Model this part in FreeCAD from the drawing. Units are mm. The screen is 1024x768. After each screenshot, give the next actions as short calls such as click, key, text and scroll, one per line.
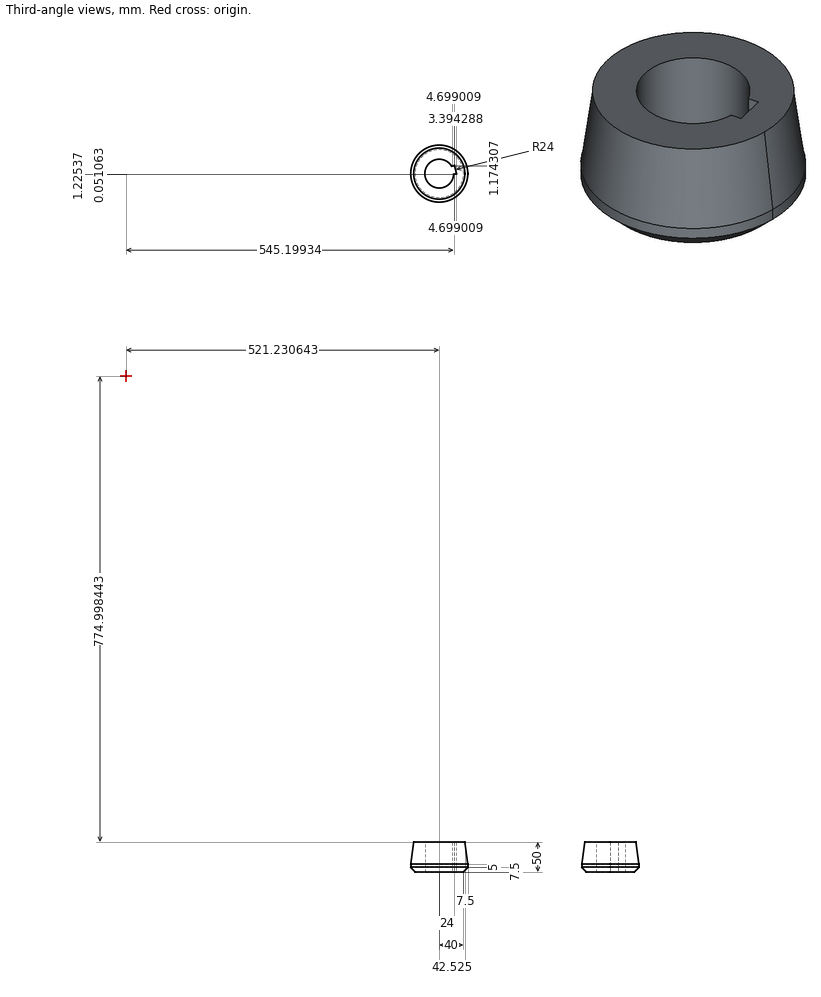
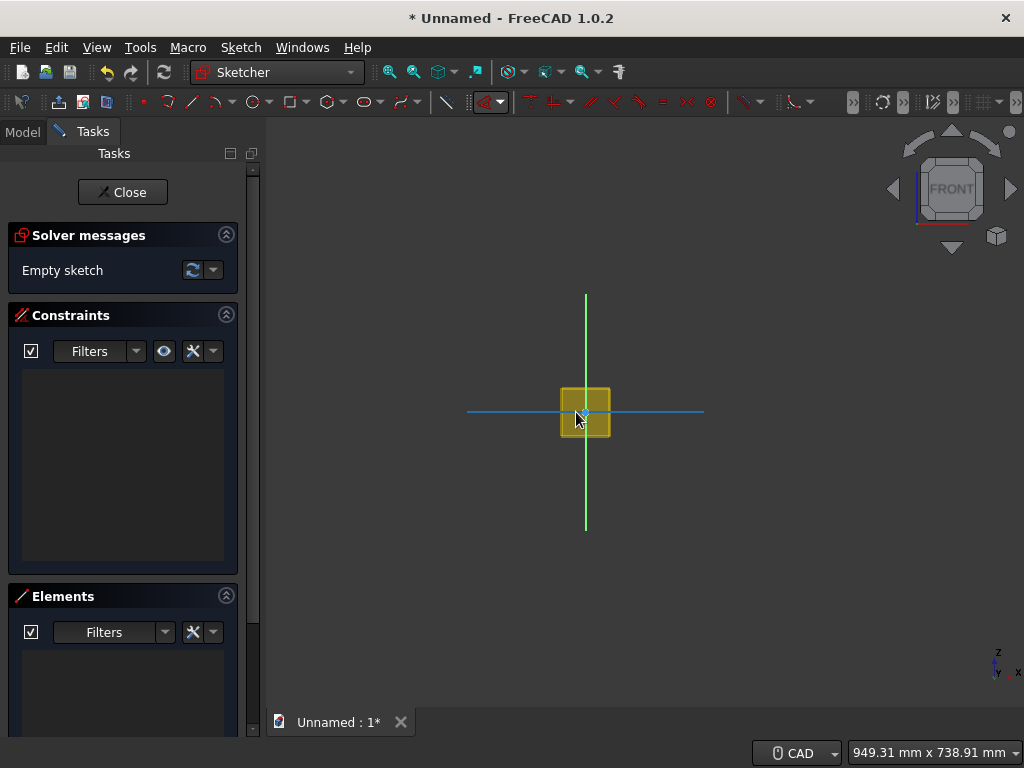
scroll(576, 412, down, 5)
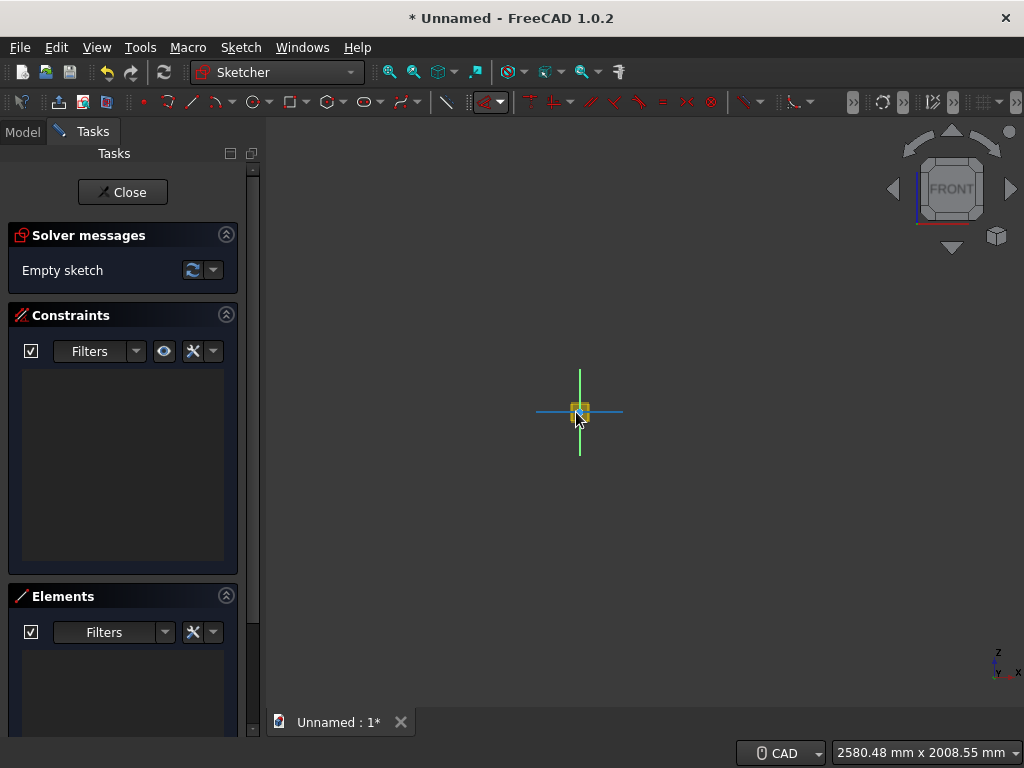
scroll(748, 657, up, 15)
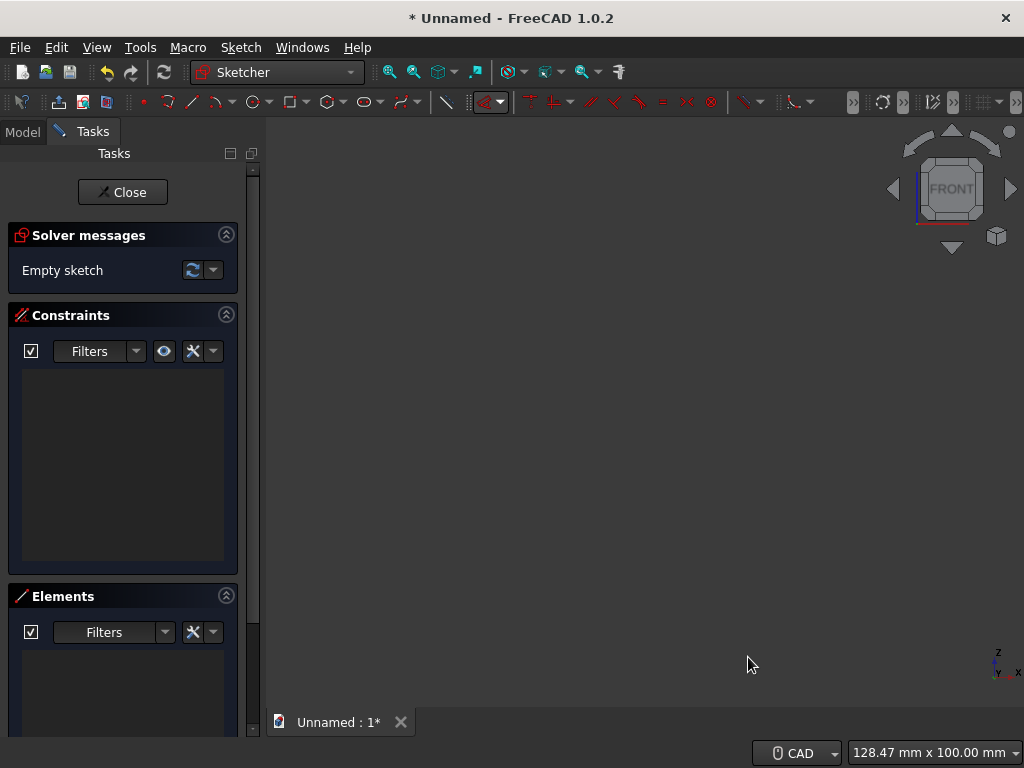
click(168, 102)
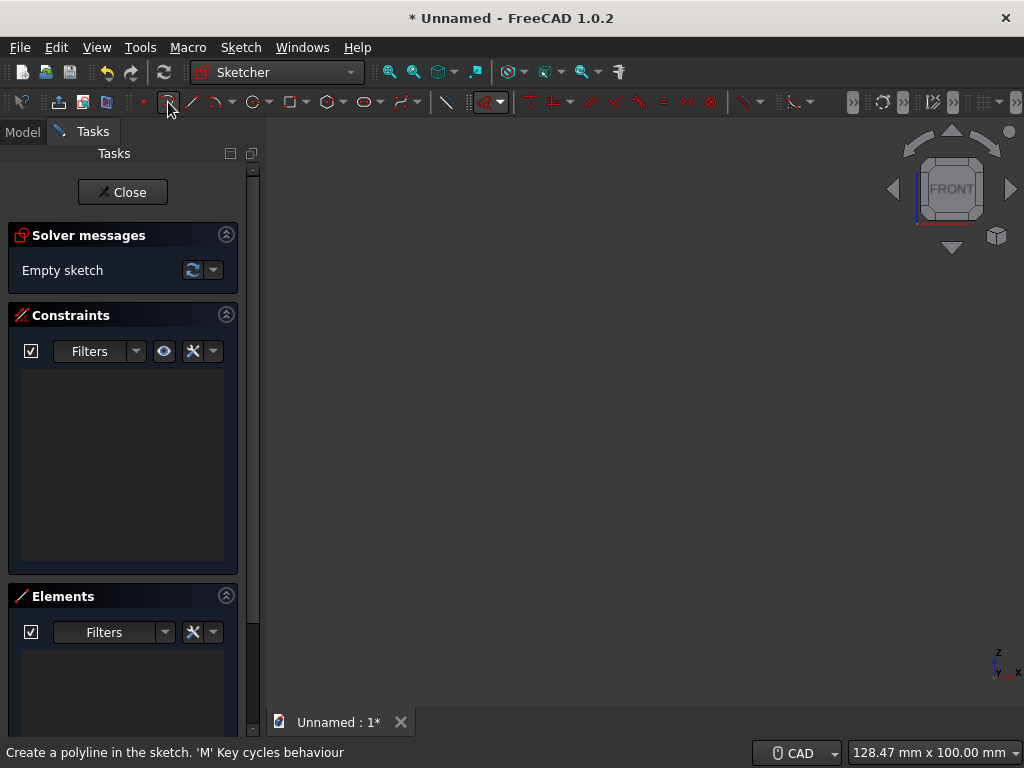
click(433, 301)
click(684, 301)
click(713, 522)
click(713, 551)
click(669, 596)
click(433, 596)
click(433, 302)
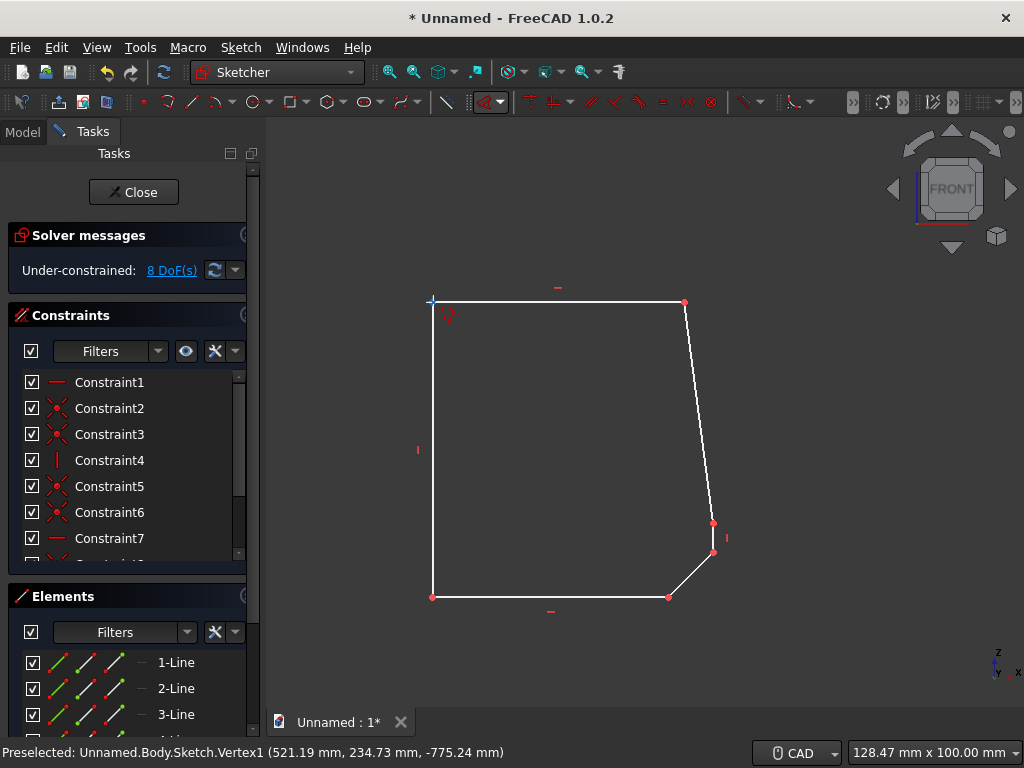
click(192, 102)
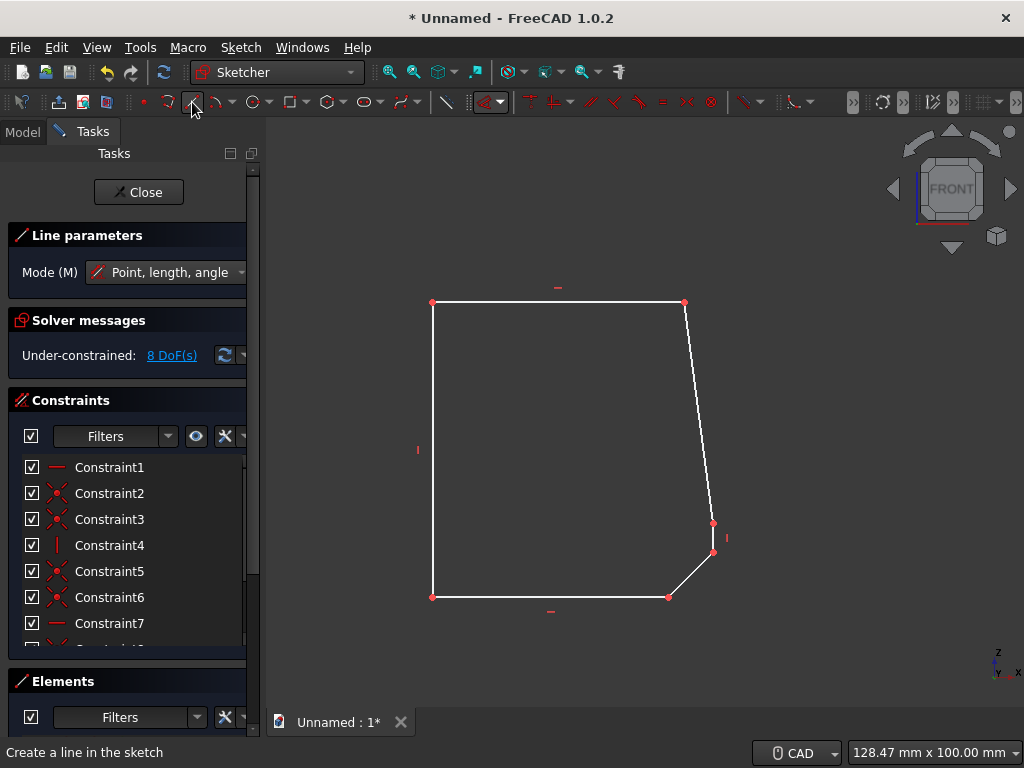
click(433, 271)
click(433, 183)
key(Escape)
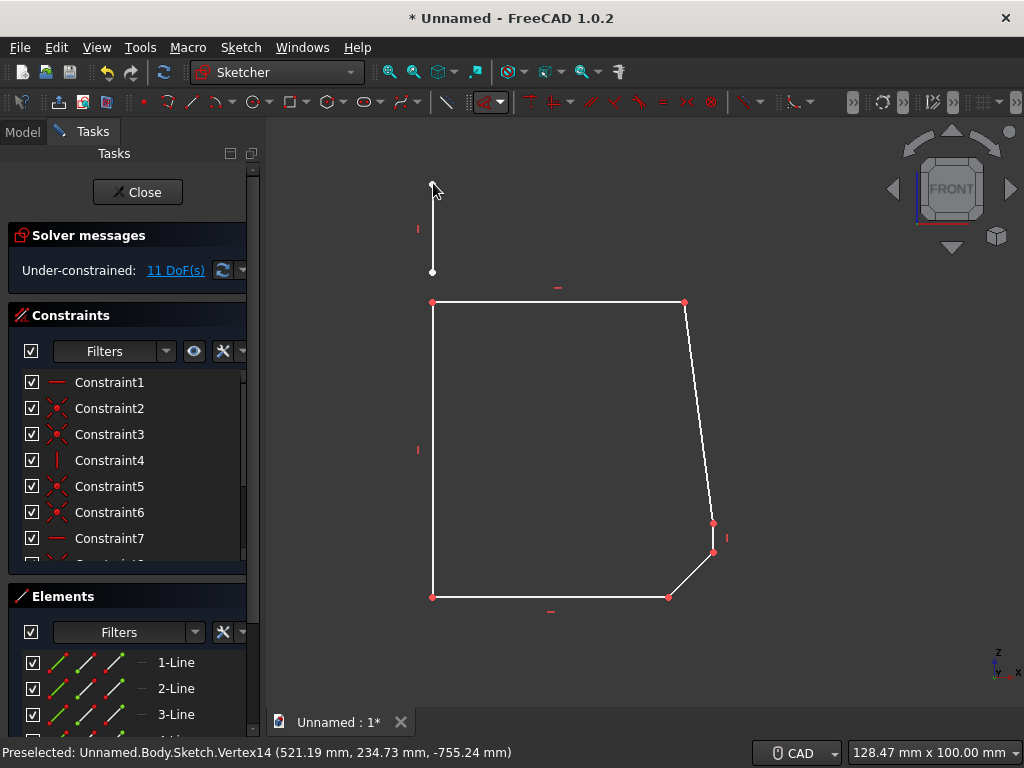
click(433, 246)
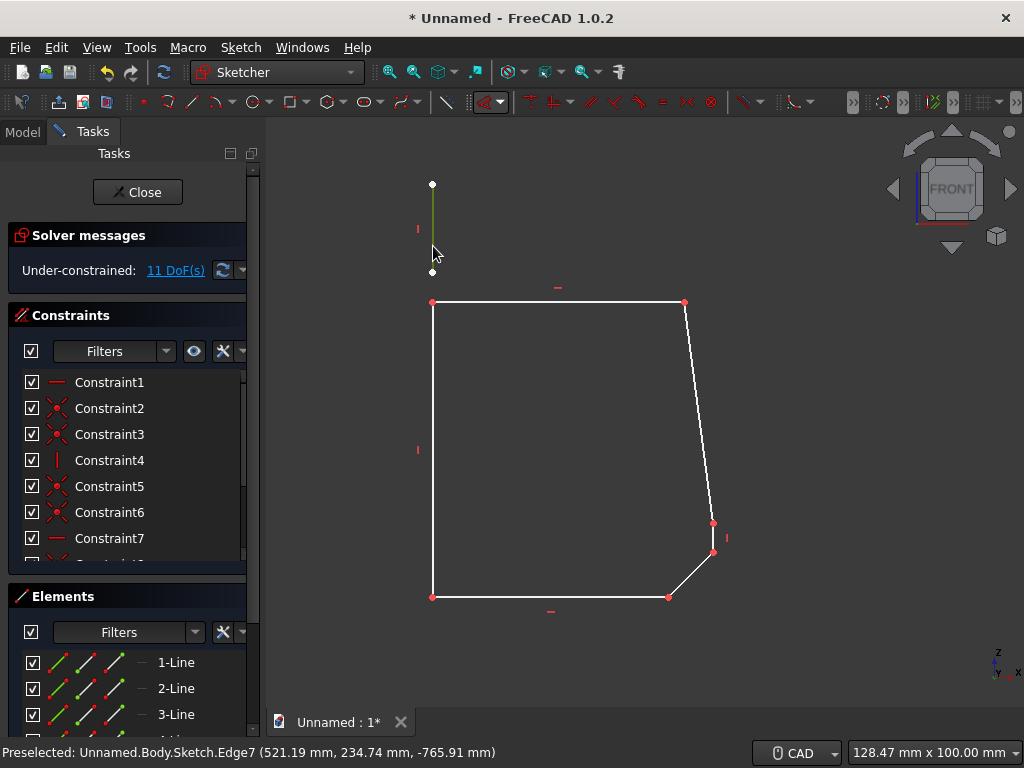
click(448, 102)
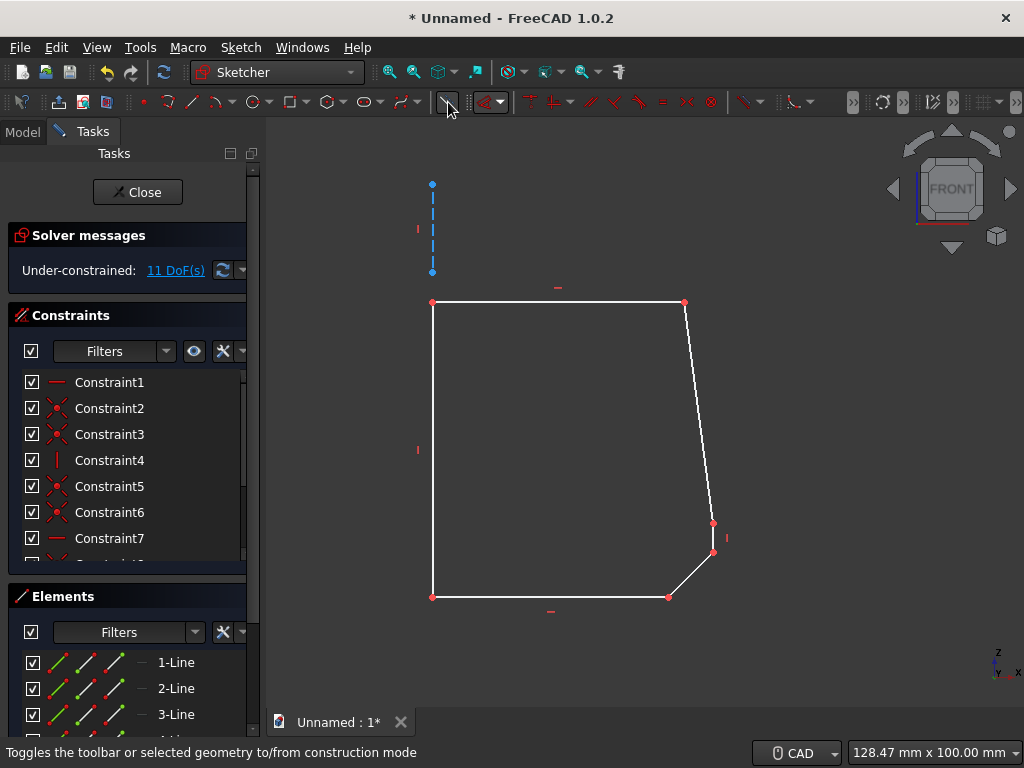
click(484, 102)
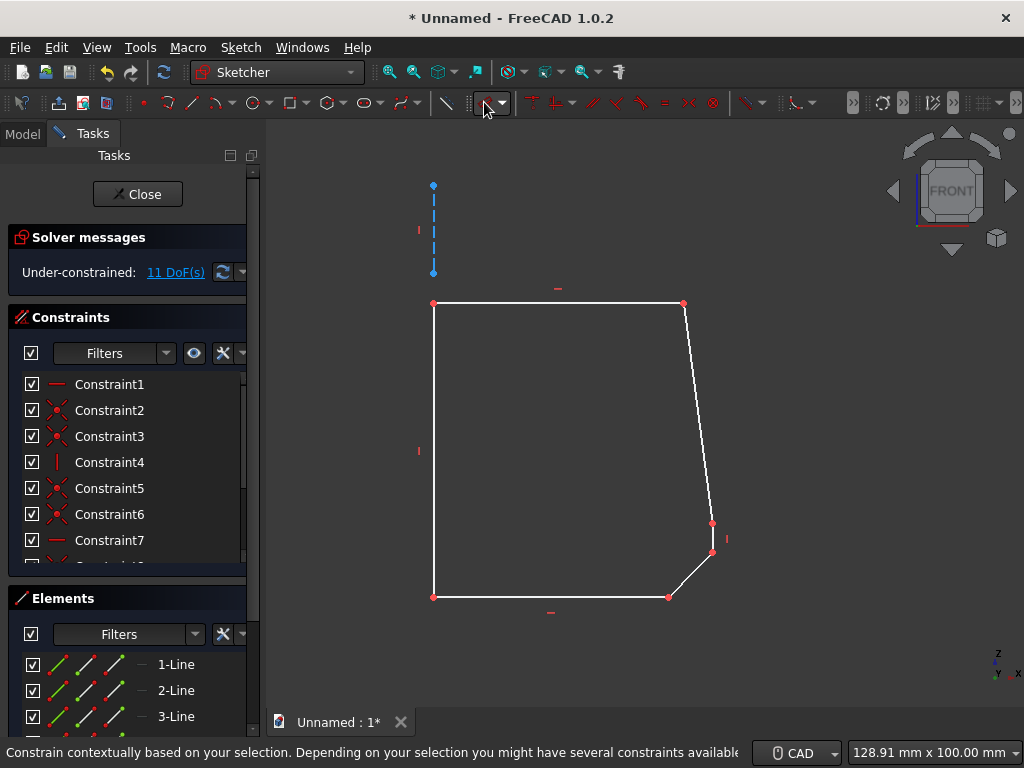
scroll(713, 535, up, 2)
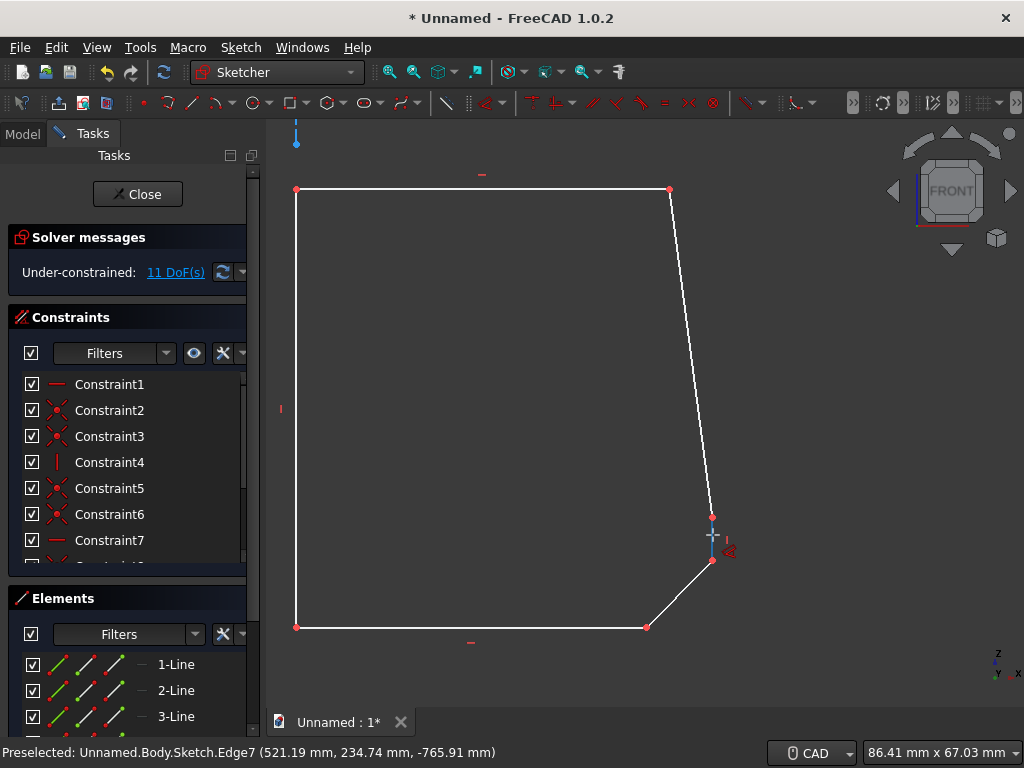
click(712, 535)
click(746, 539)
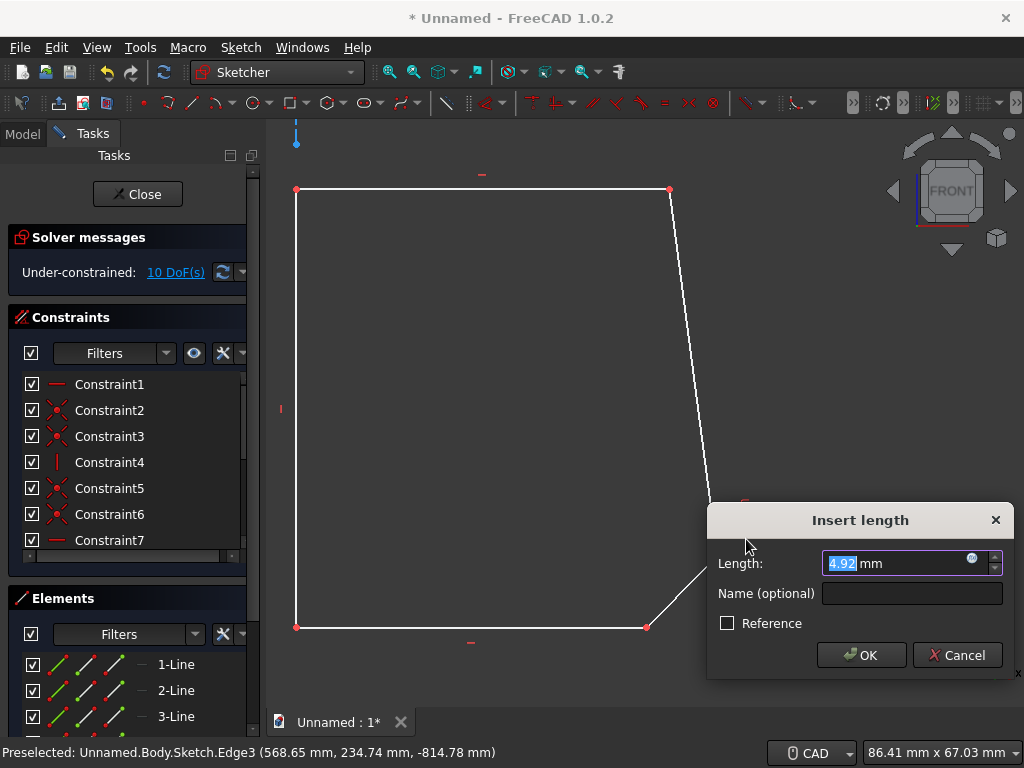
text(5)
key(Return)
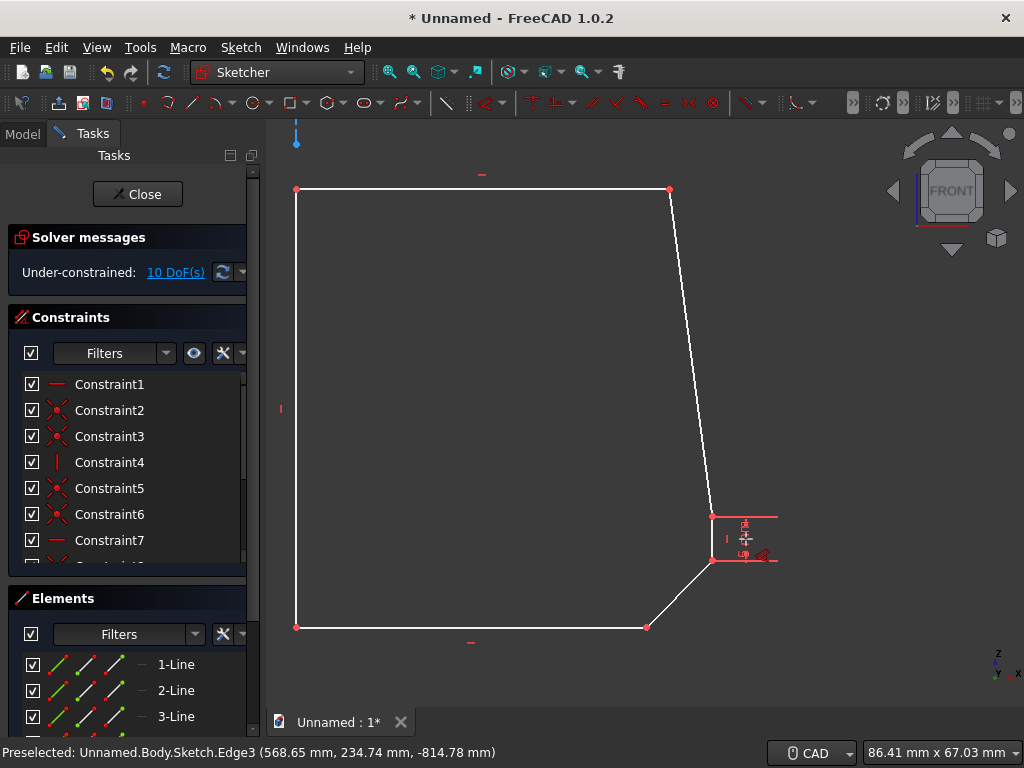
click(542, 628)
click(472, 662)